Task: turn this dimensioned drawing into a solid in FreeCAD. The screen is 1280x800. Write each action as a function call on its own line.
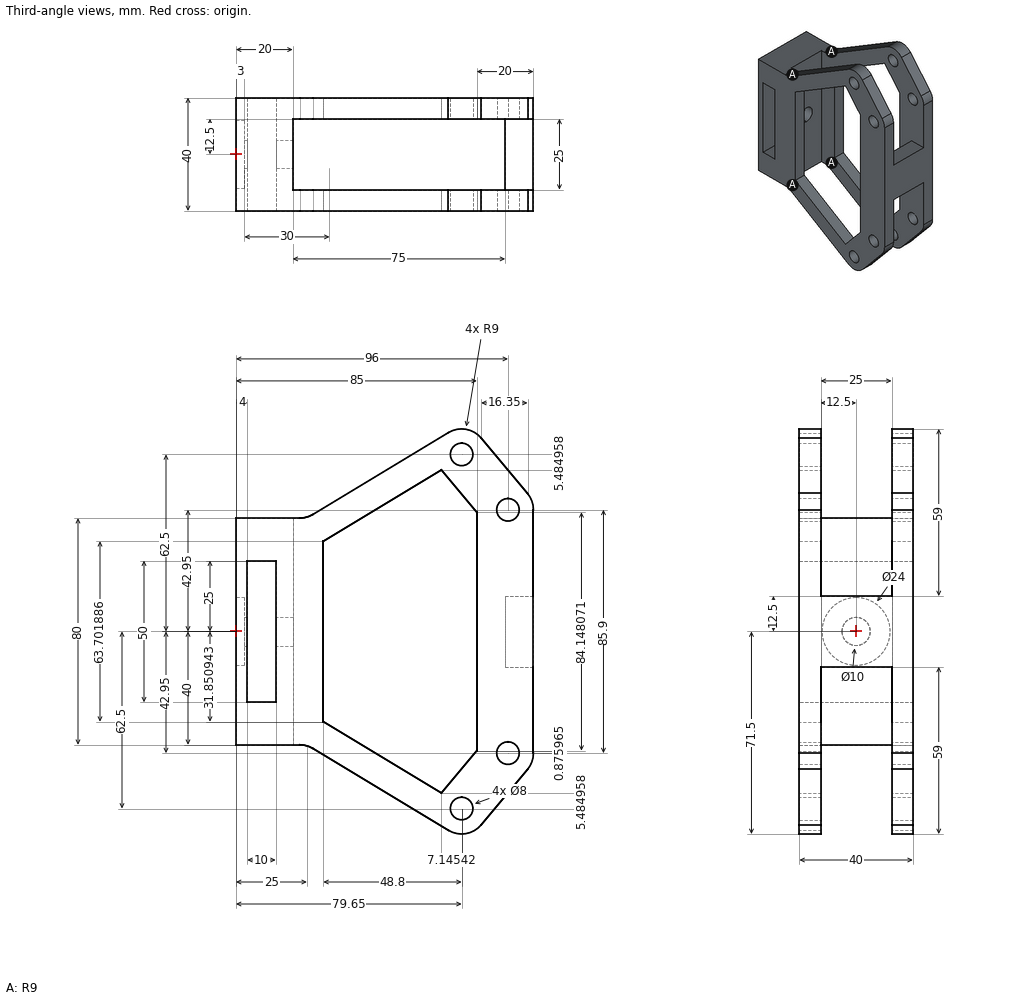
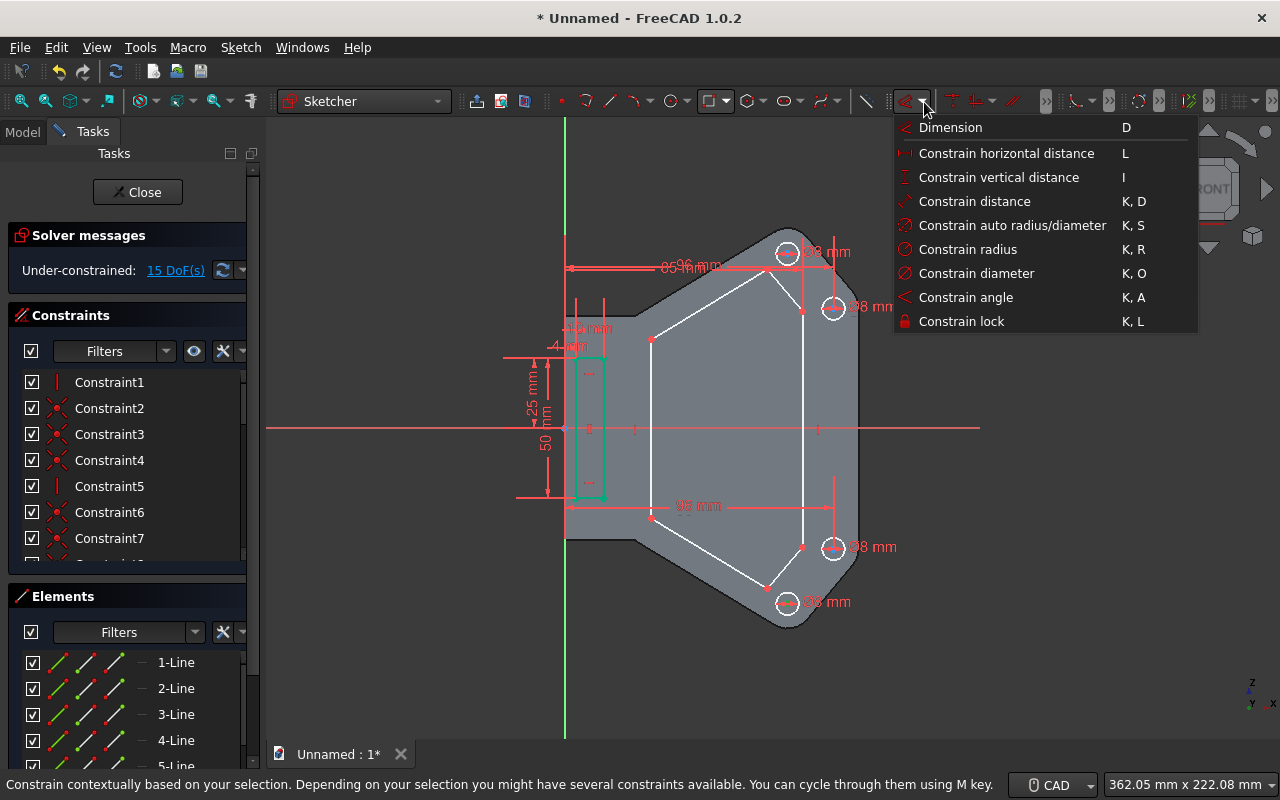
click(1046, 177)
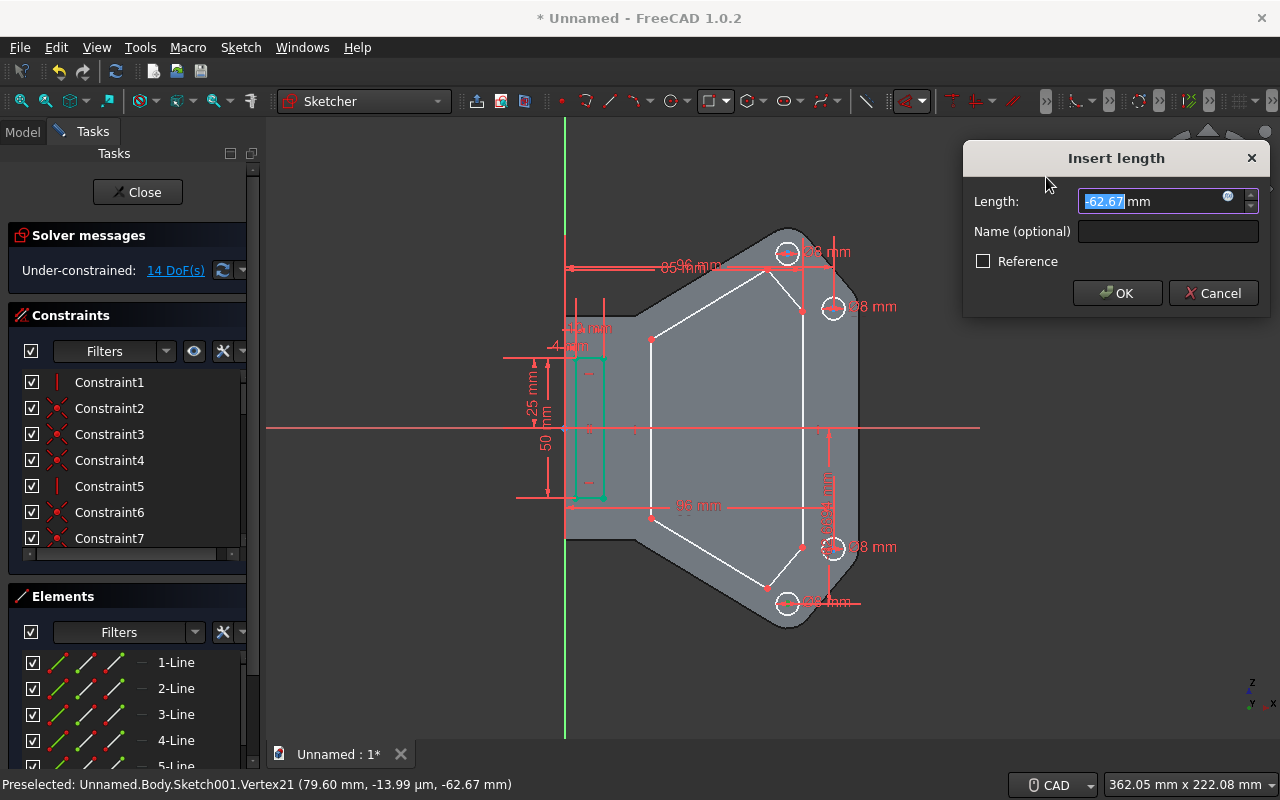
text(-62.5)
key(Return)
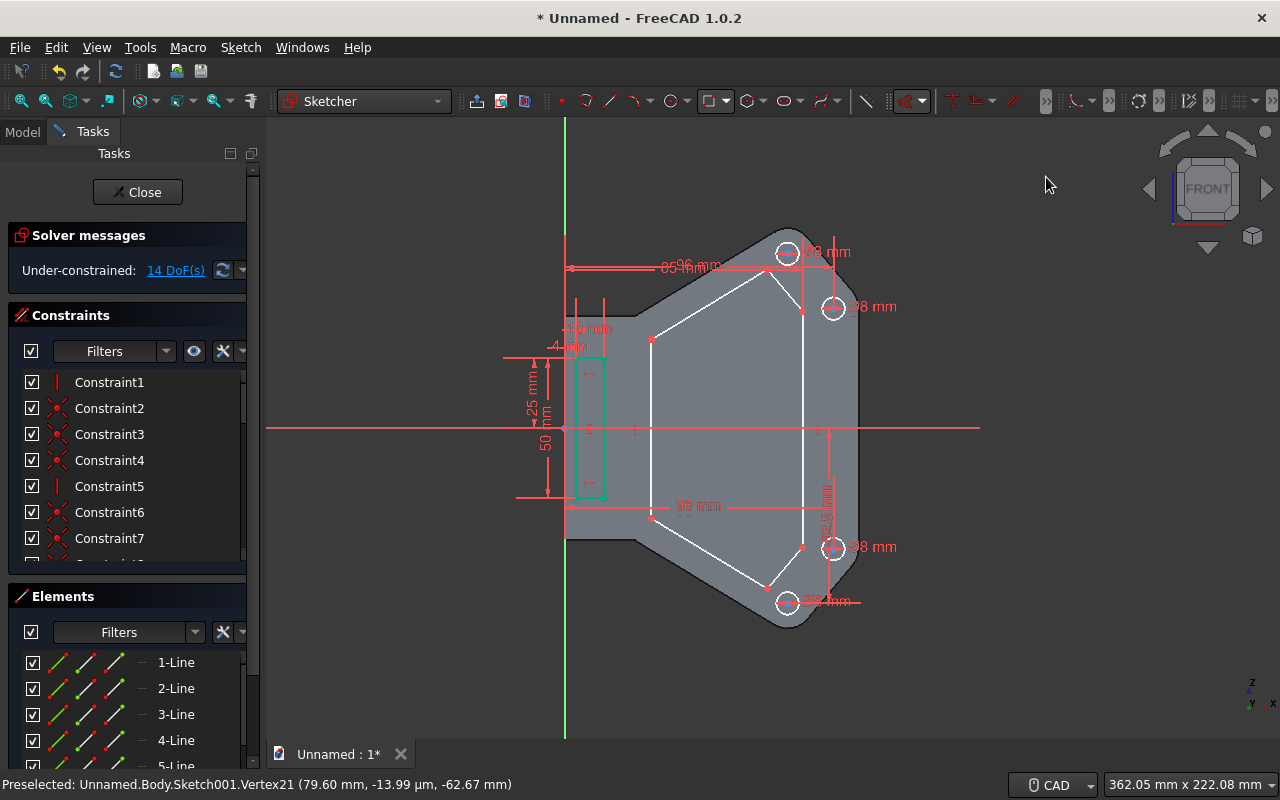
click(788, 254)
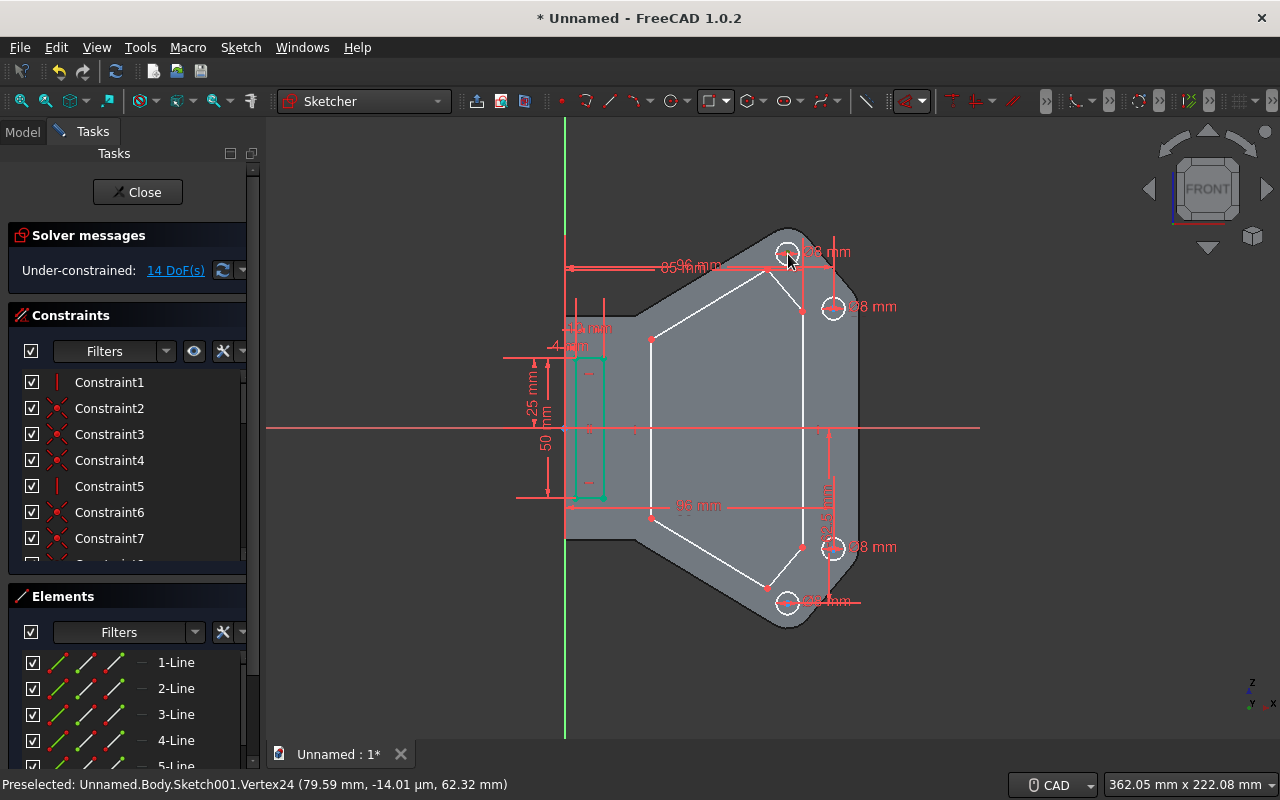
key(i)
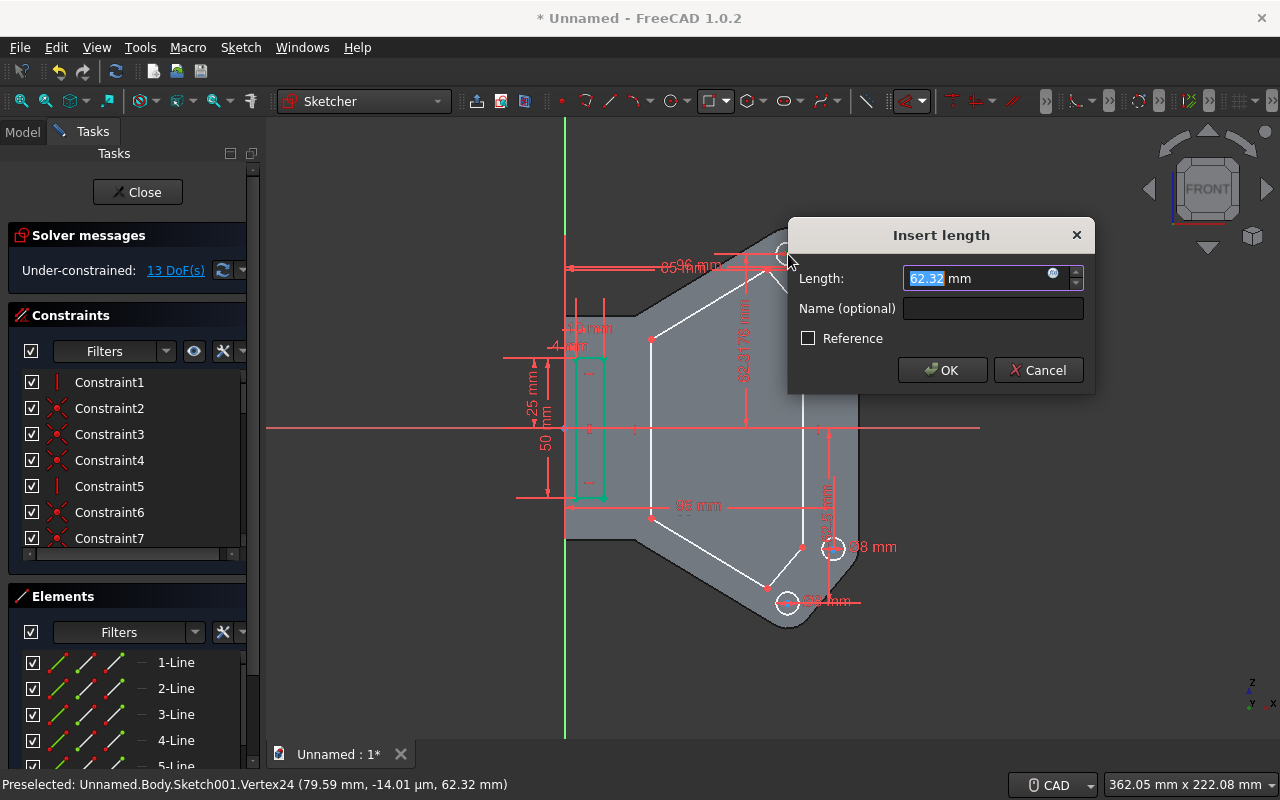
text(62.5)
key(Return)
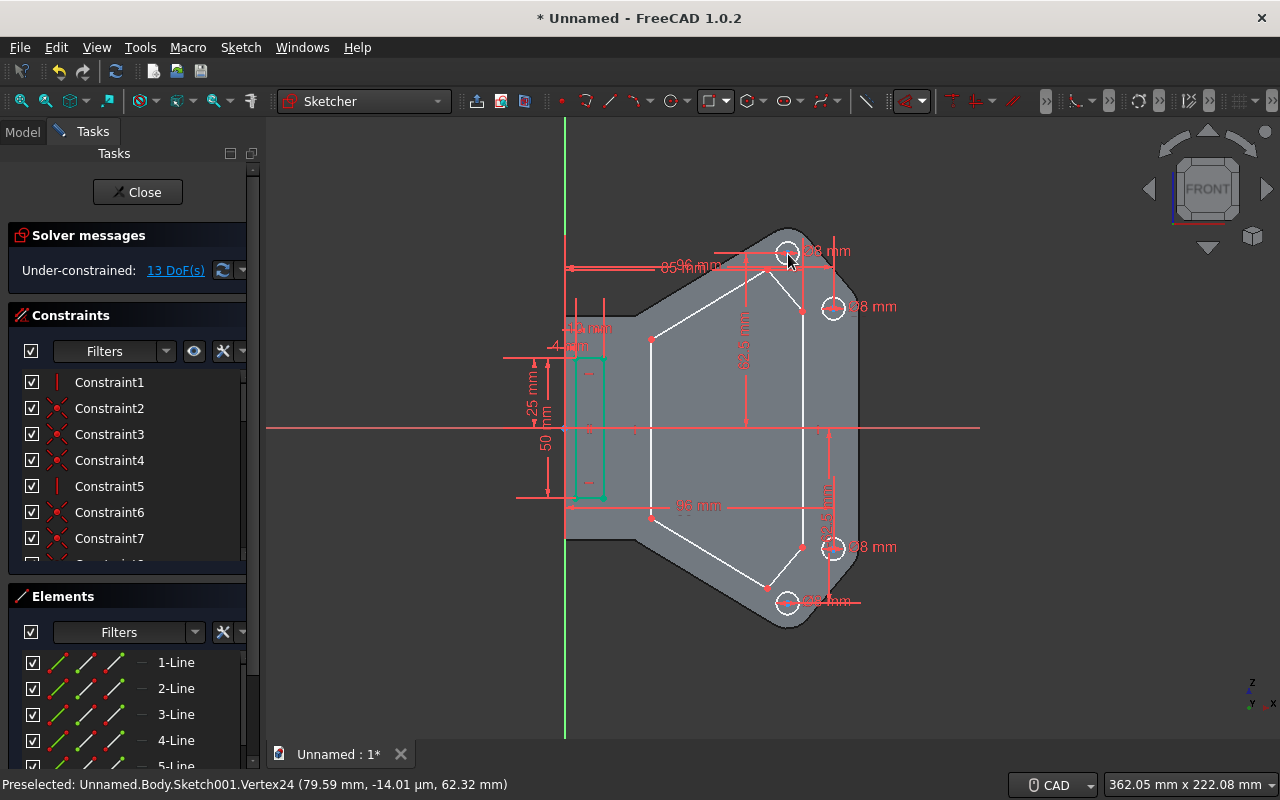
click(788, 603)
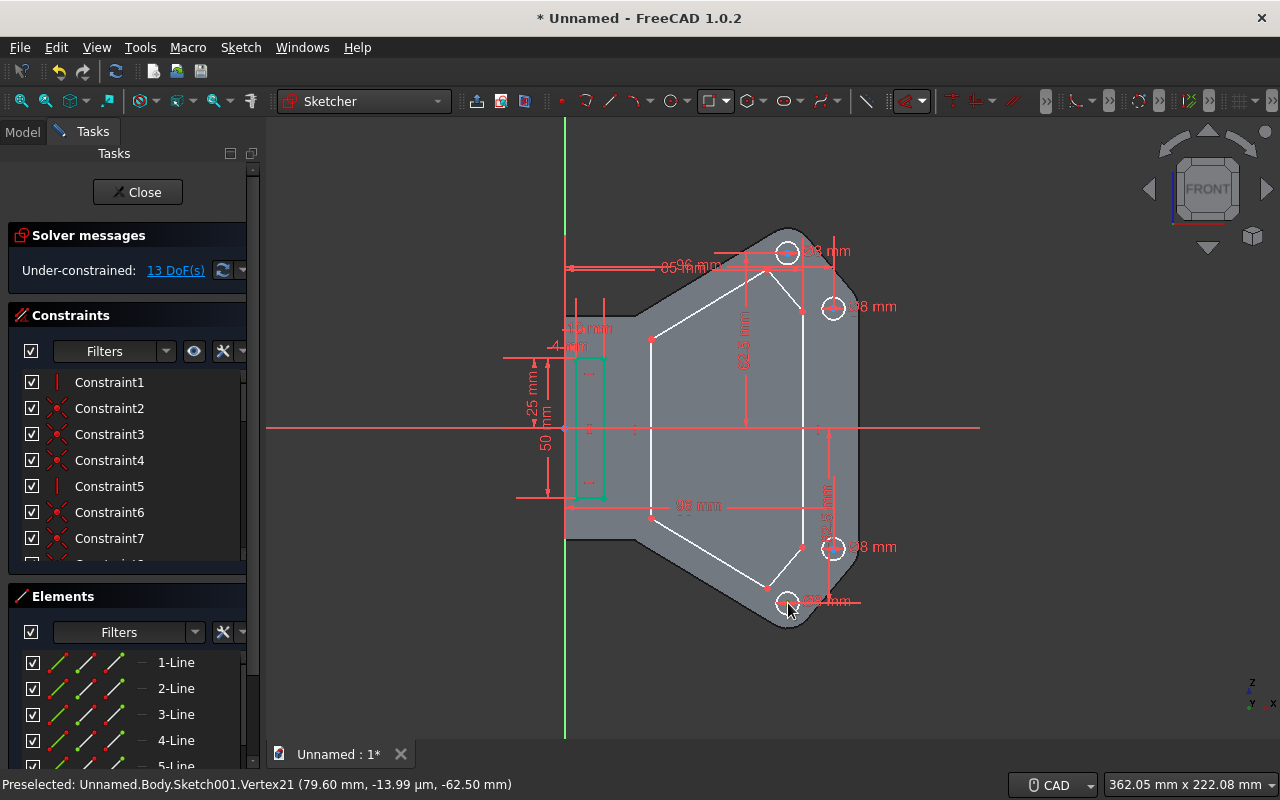
click(924, 102)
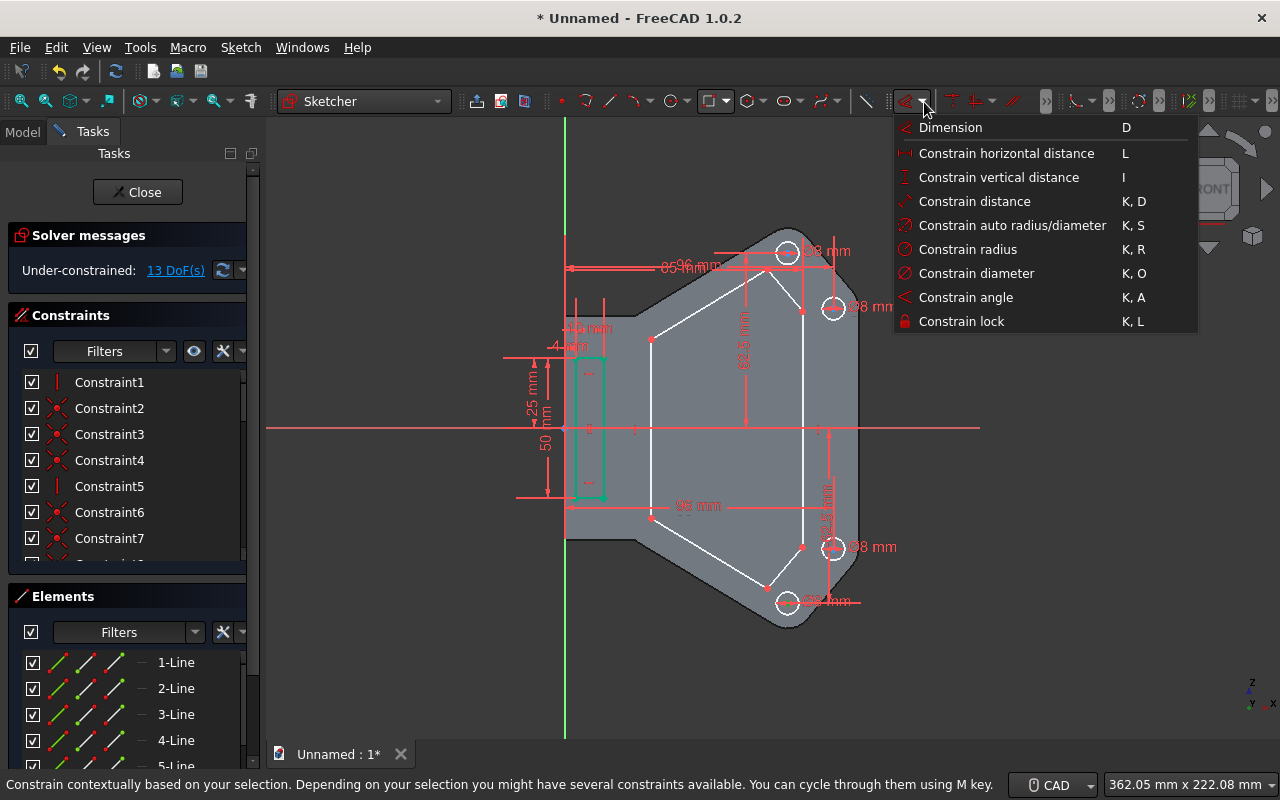
click(1046, 153)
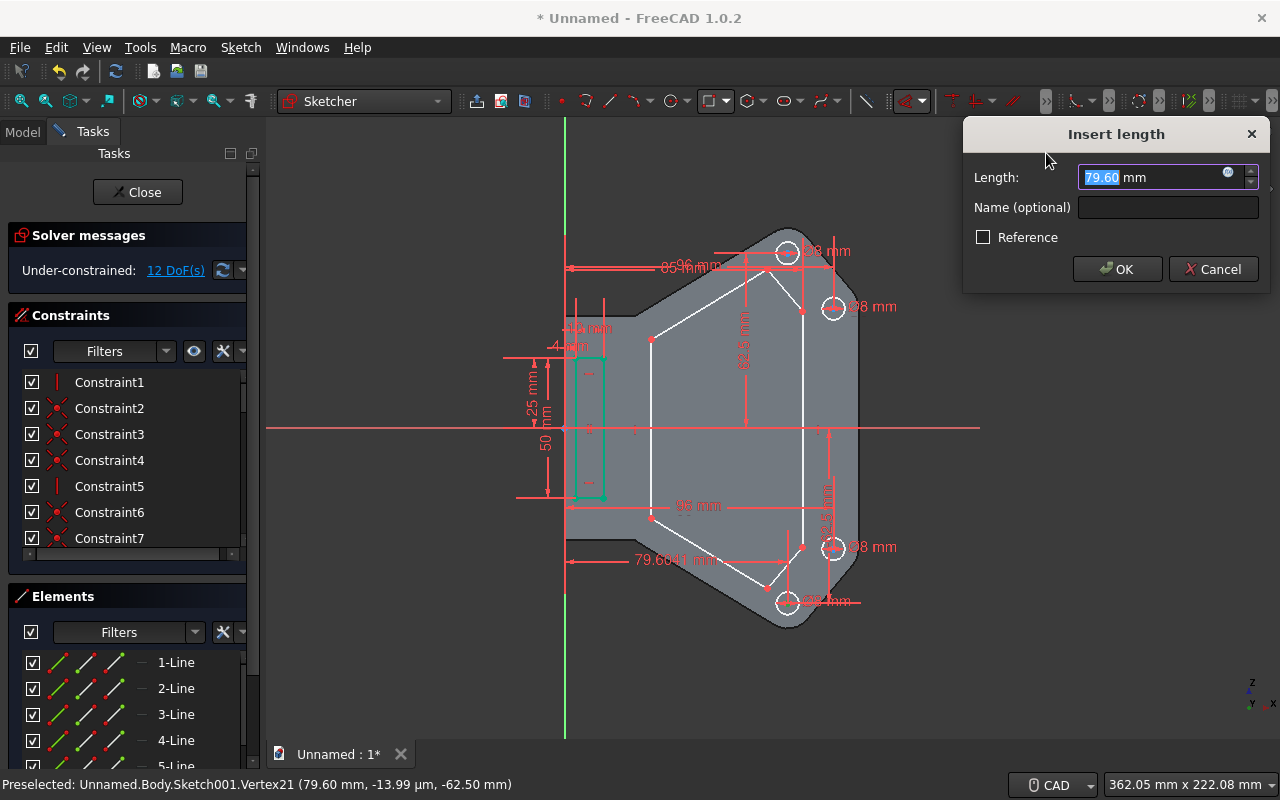
text(79.65)
key(Return)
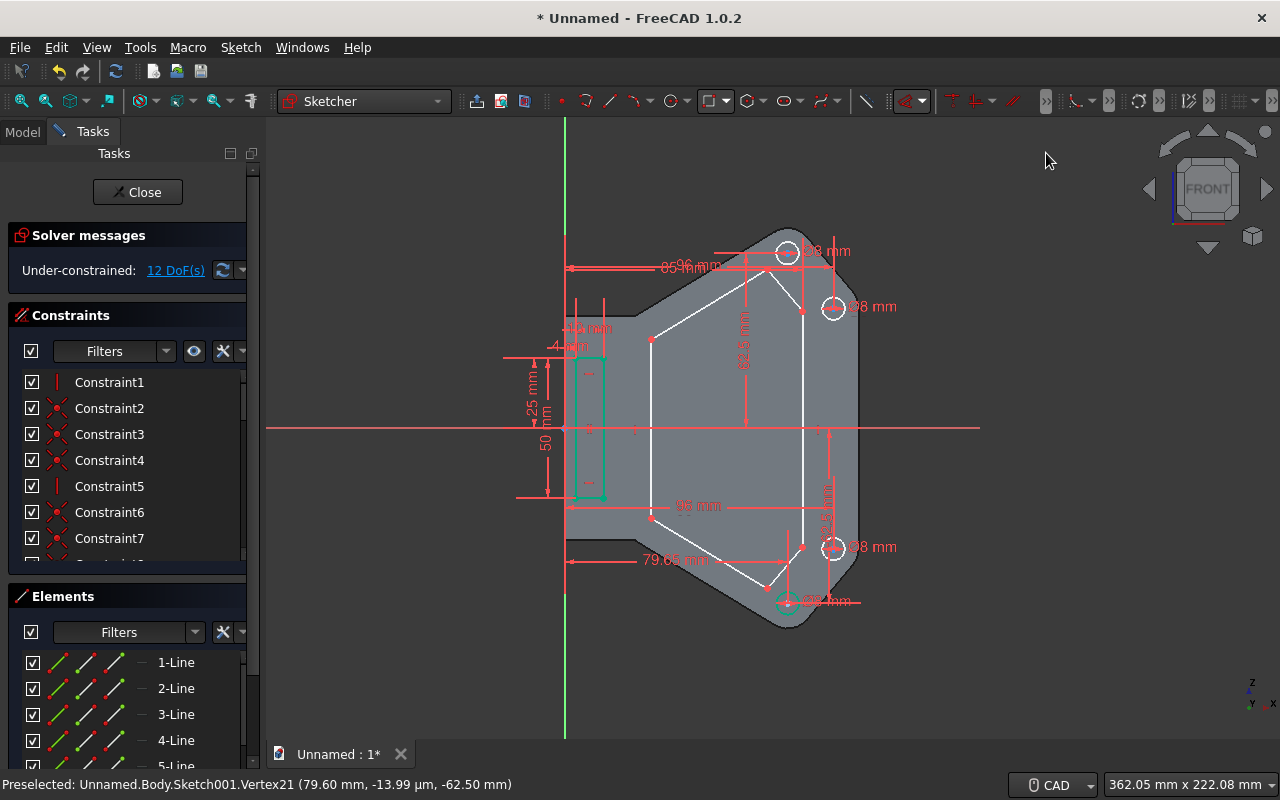
click(834, 549)